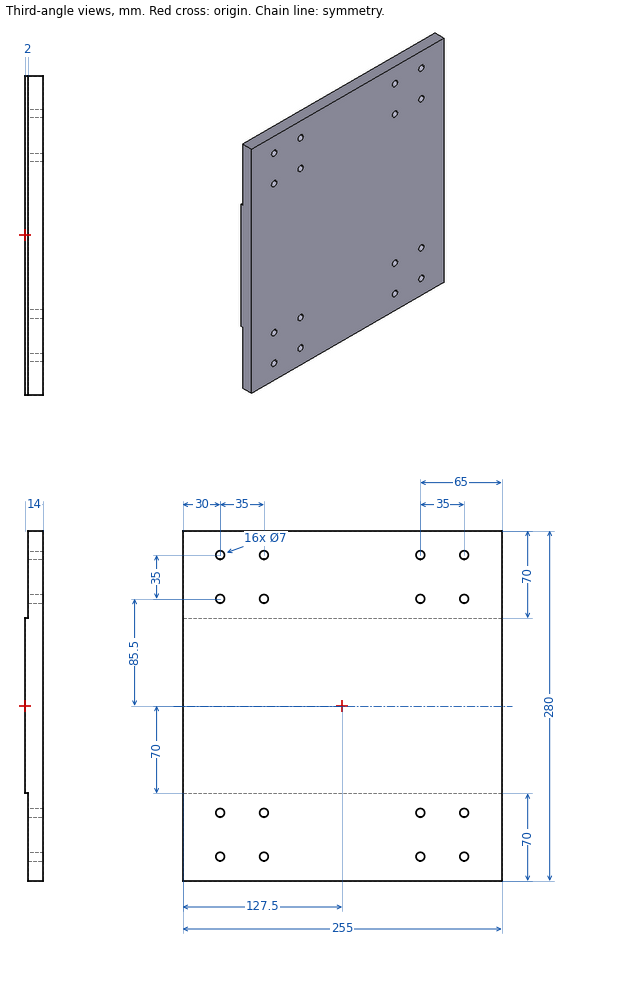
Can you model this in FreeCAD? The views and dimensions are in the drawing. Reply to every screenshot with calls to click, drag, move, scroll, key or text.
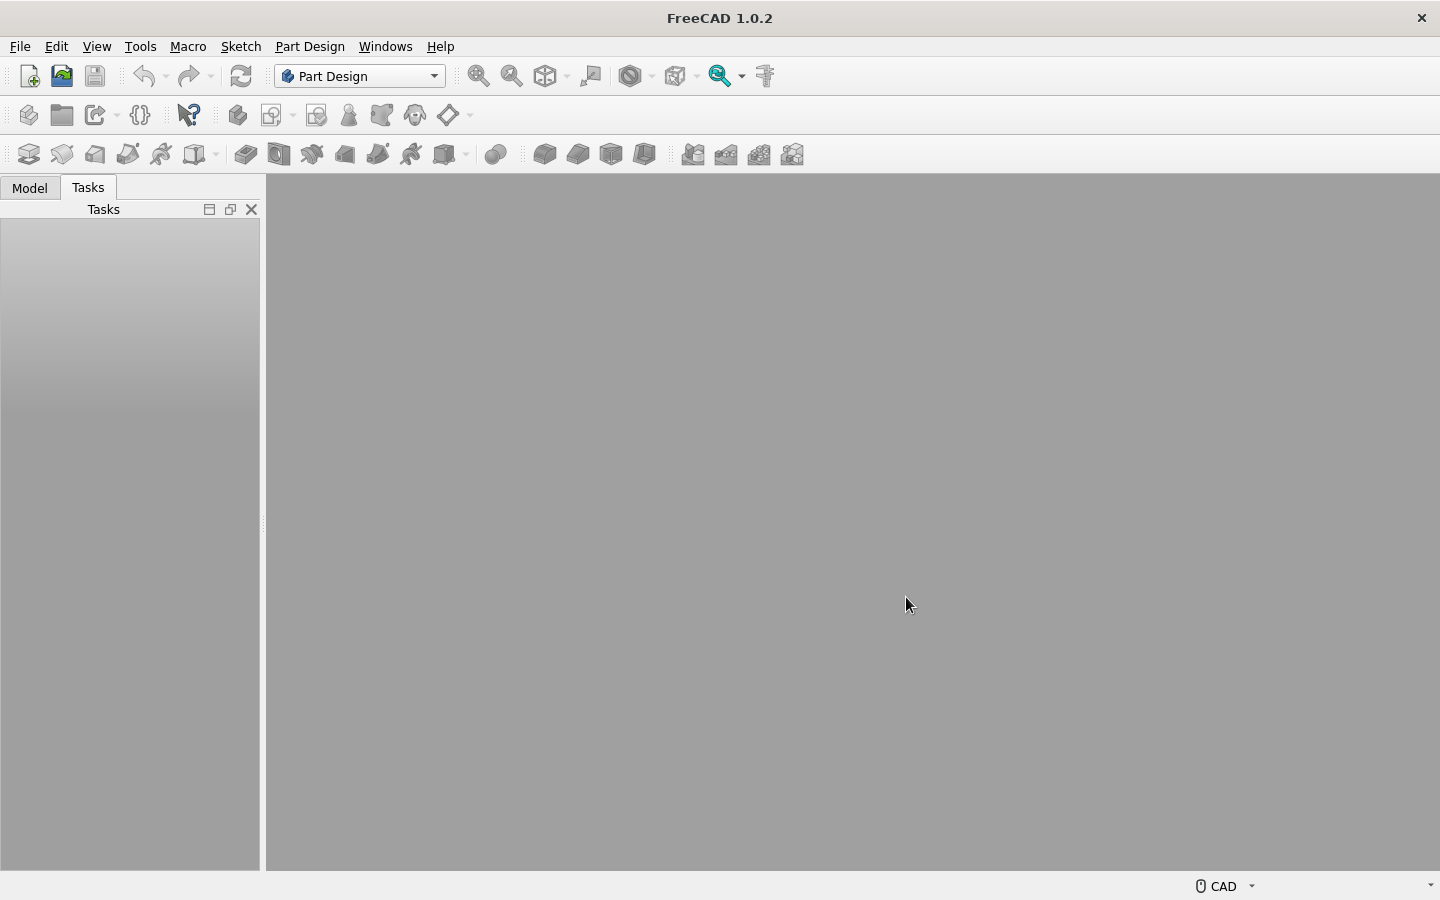
click(29, 76)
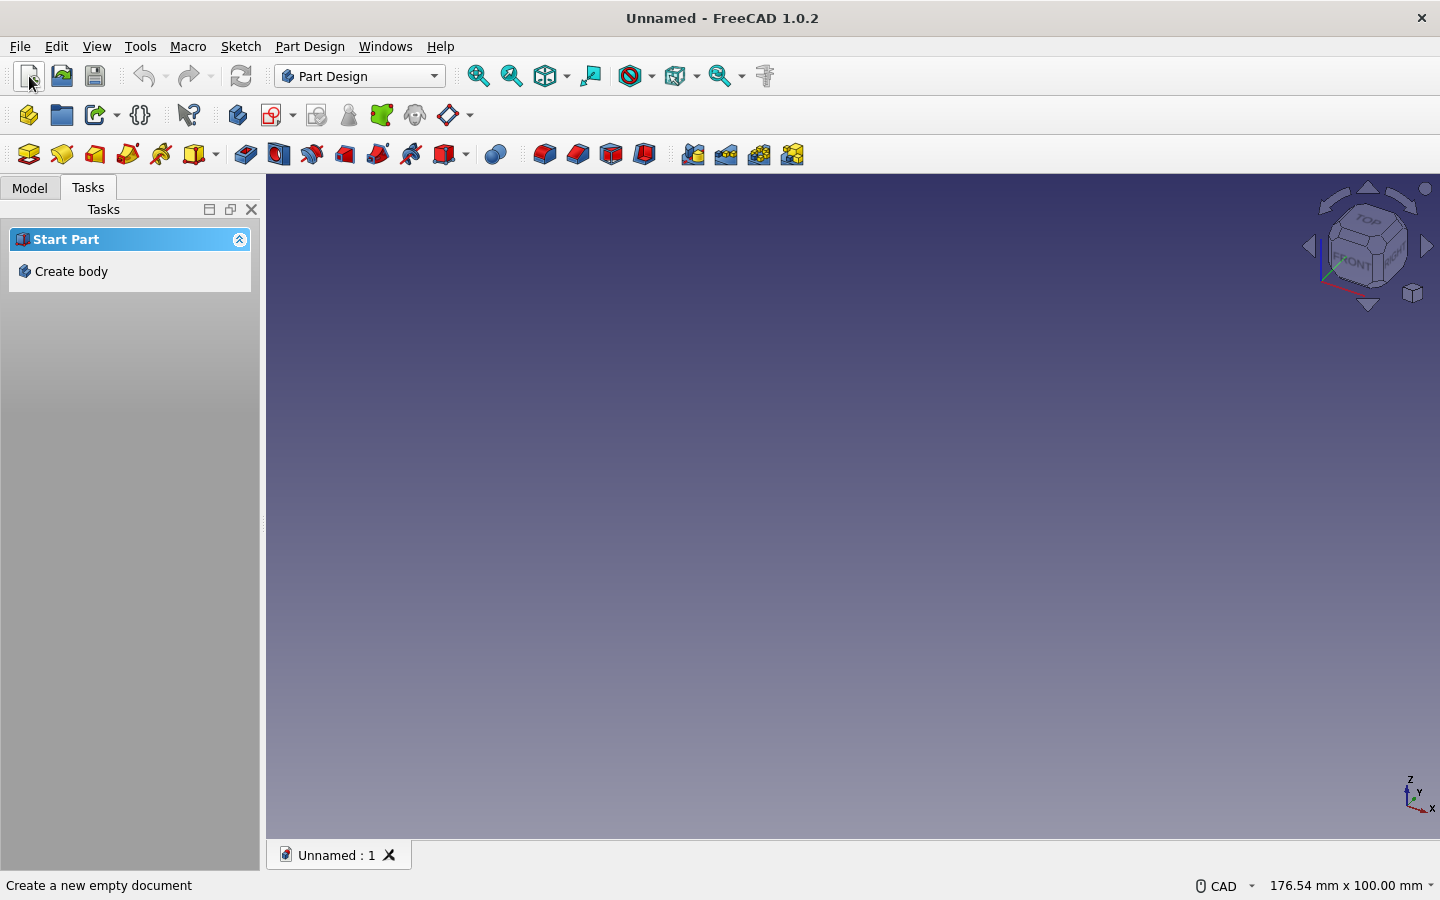
click(270, 116)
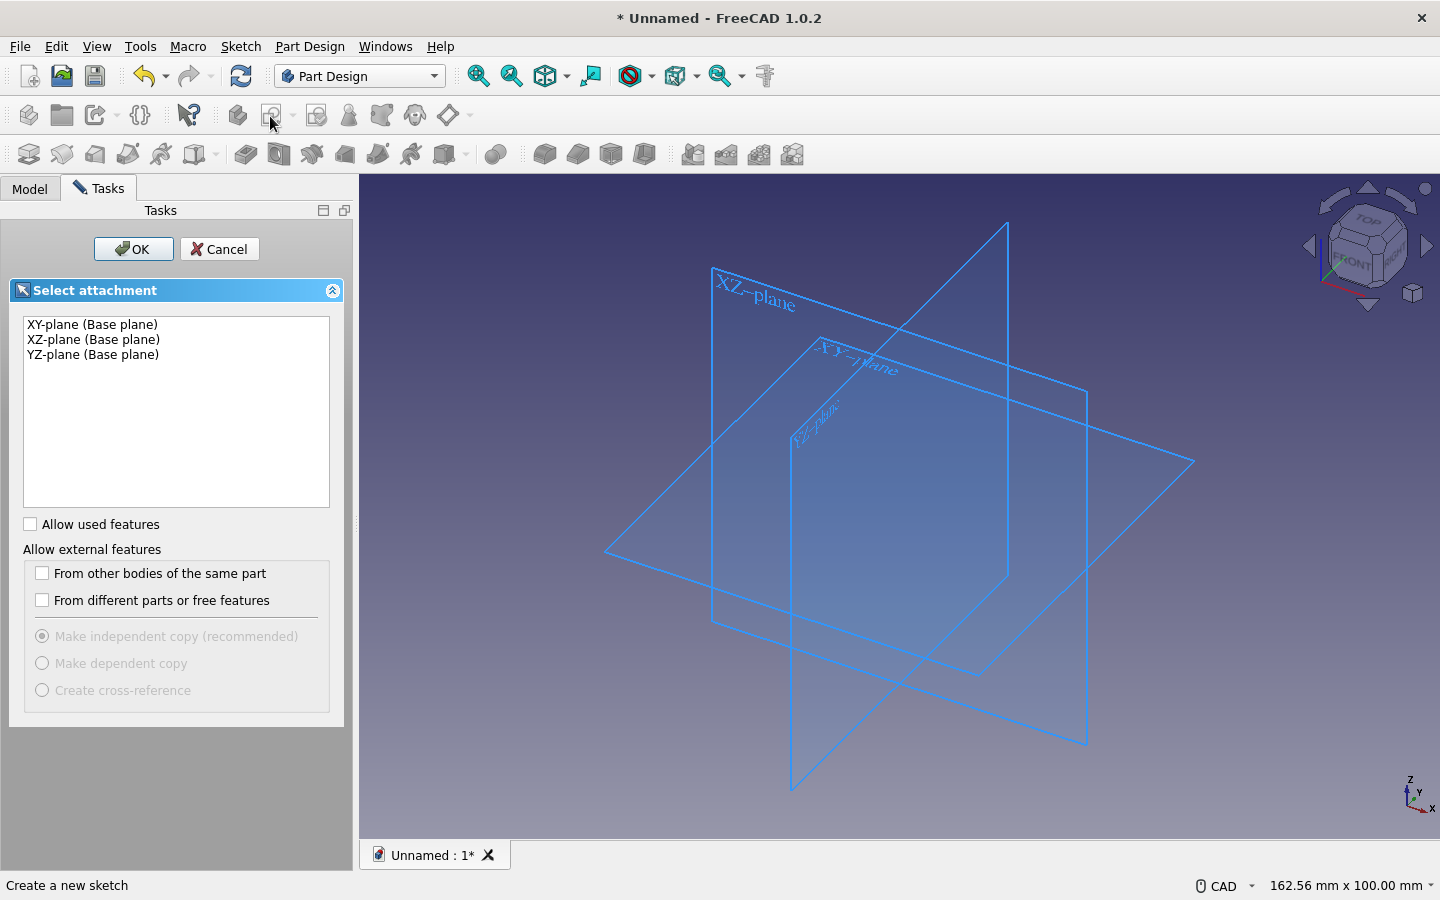
click(84, 354)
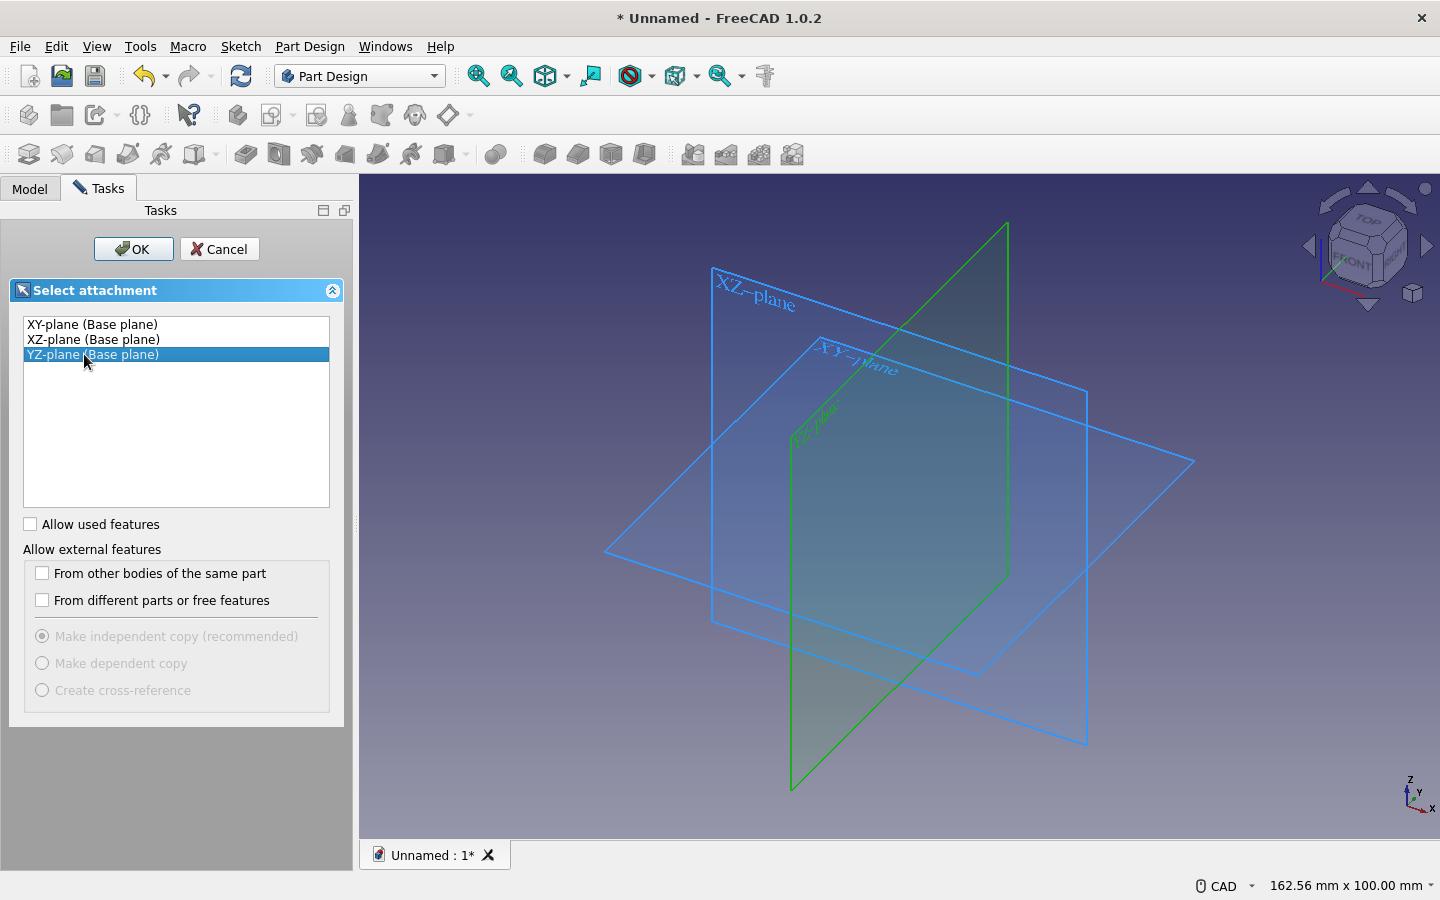
click(134, 249)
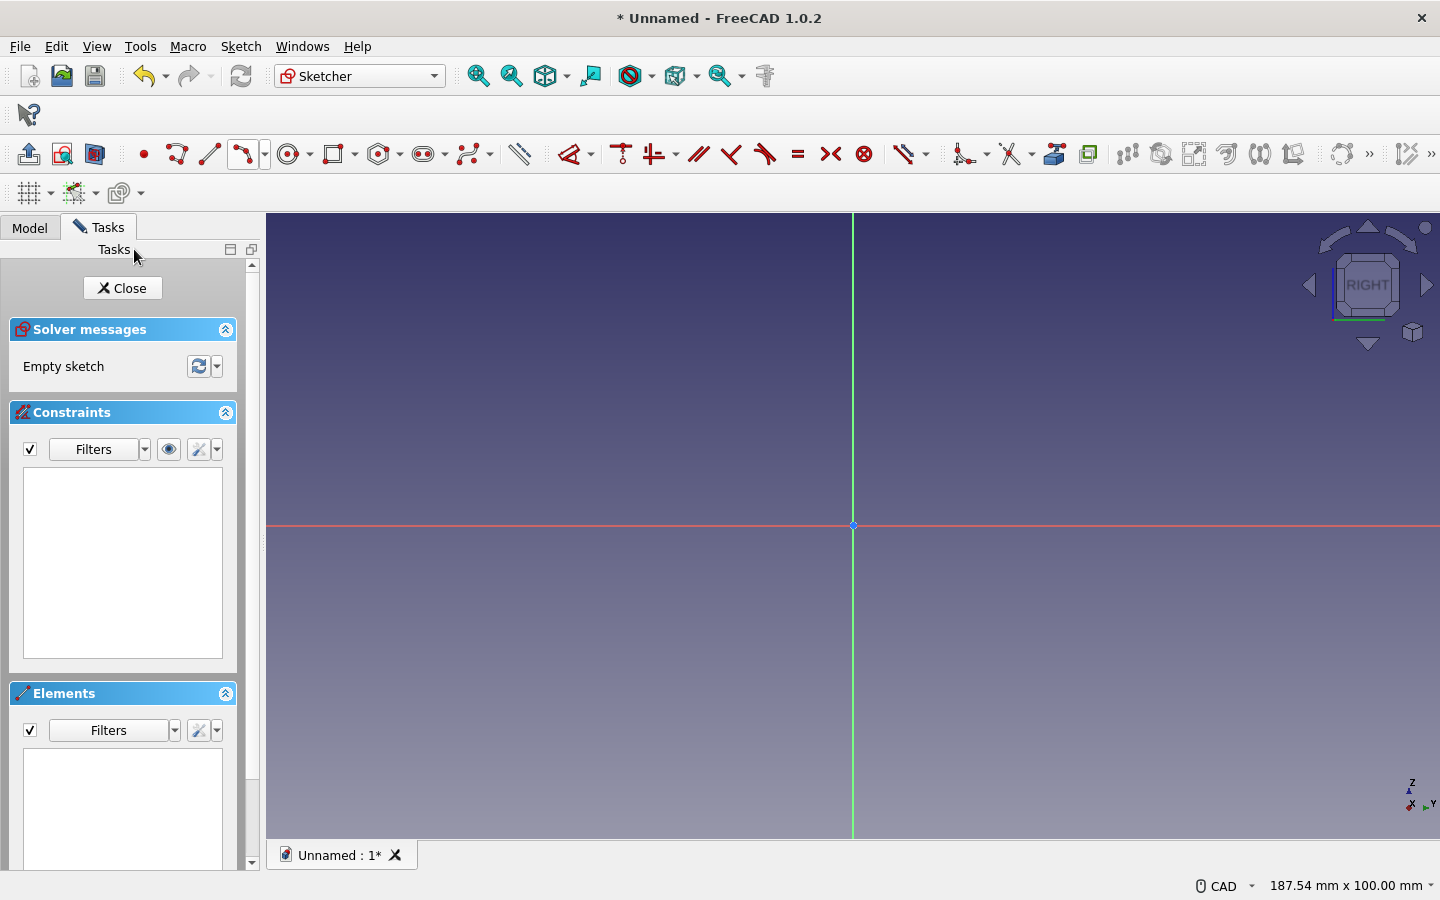
scroll(762, 526, down, 7)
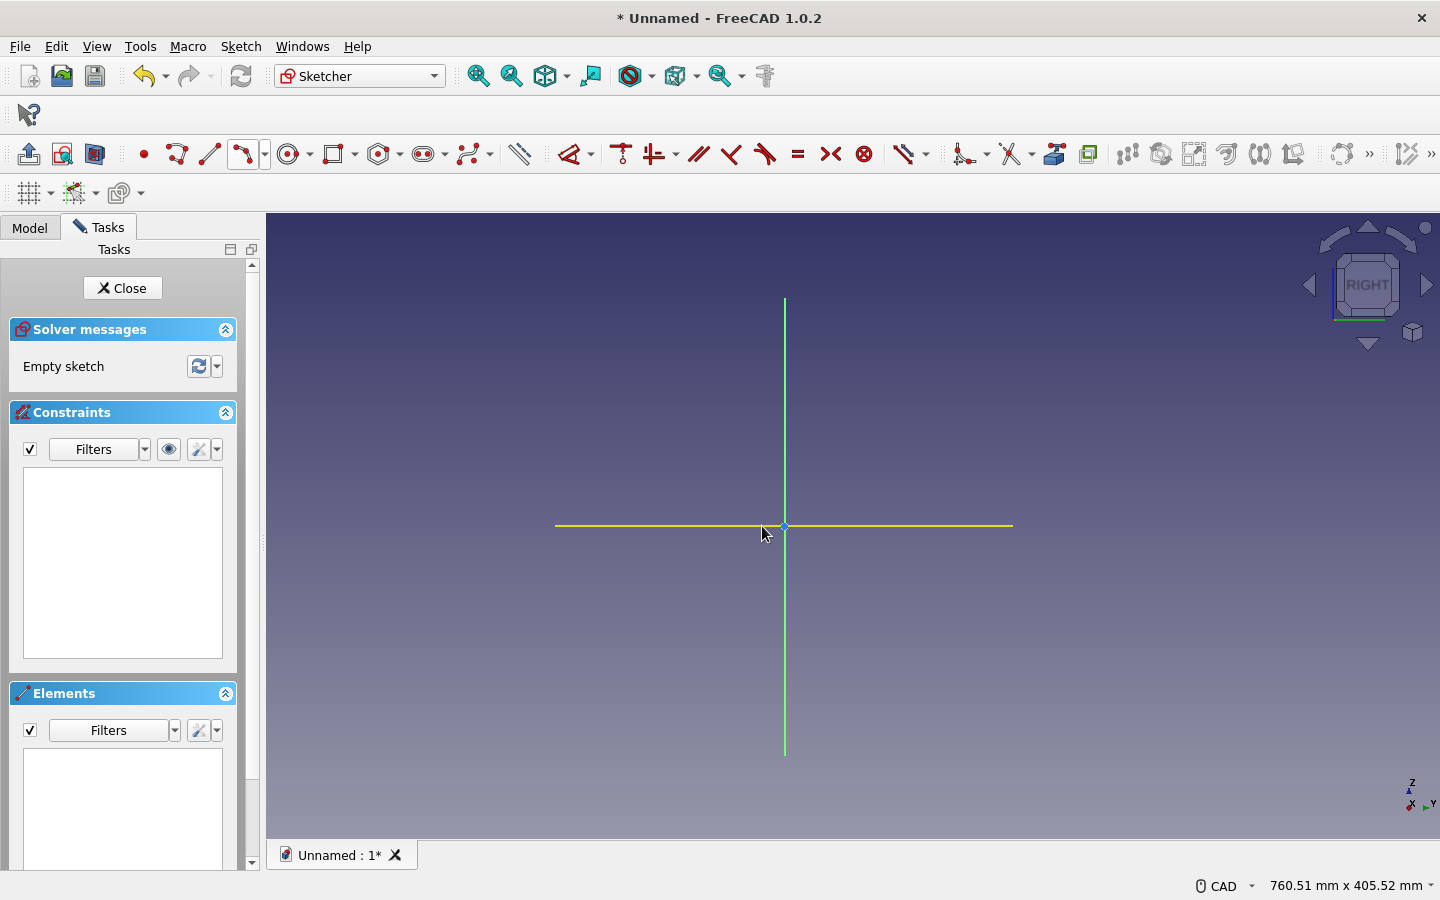
click(354, 154)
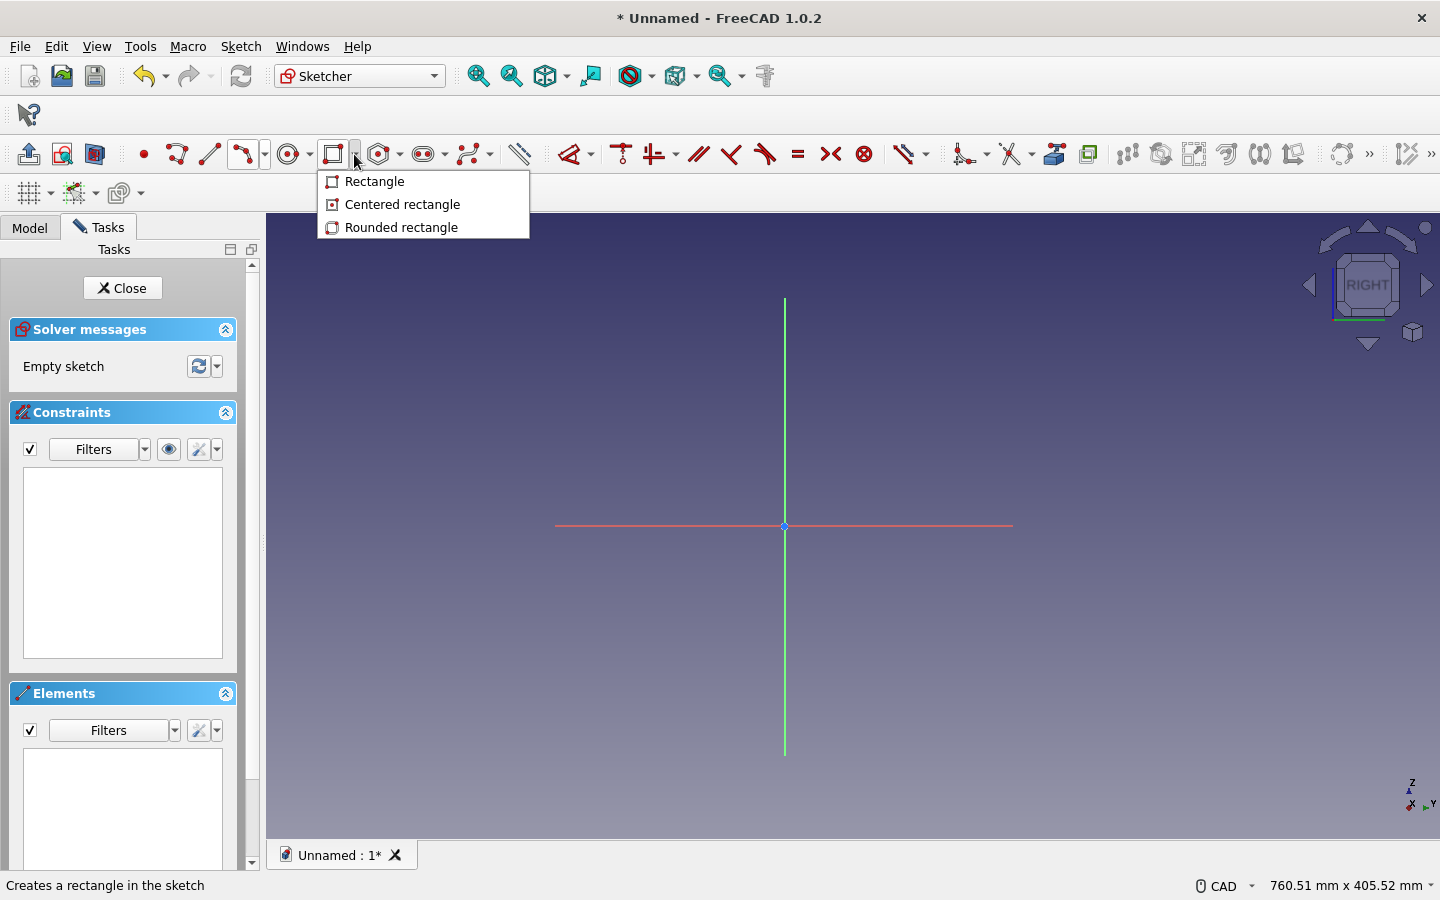
click(424, 204)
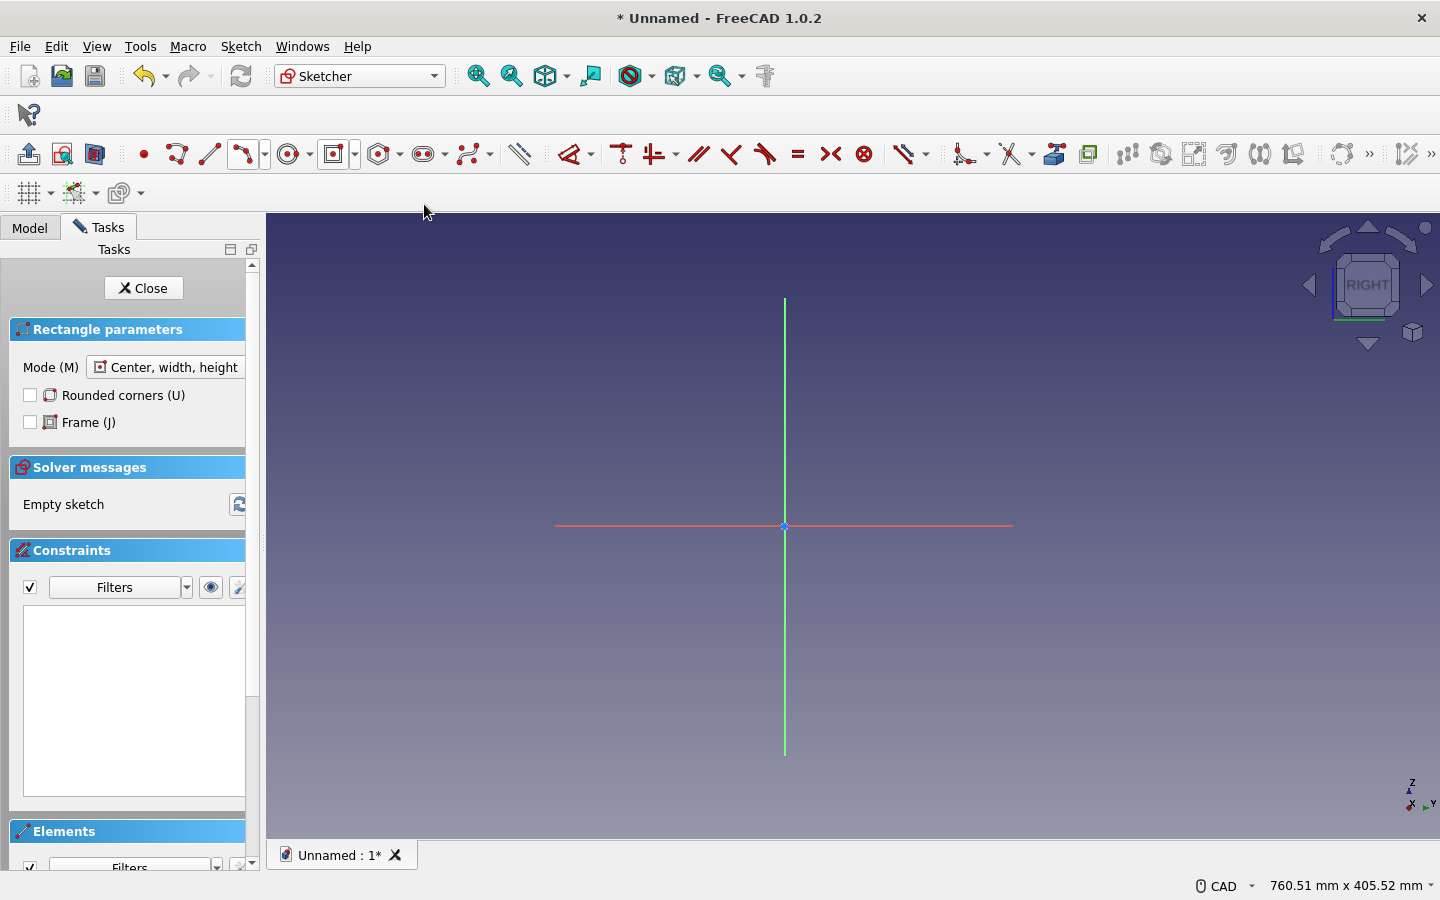
click(785, 526)
move(982, 310)